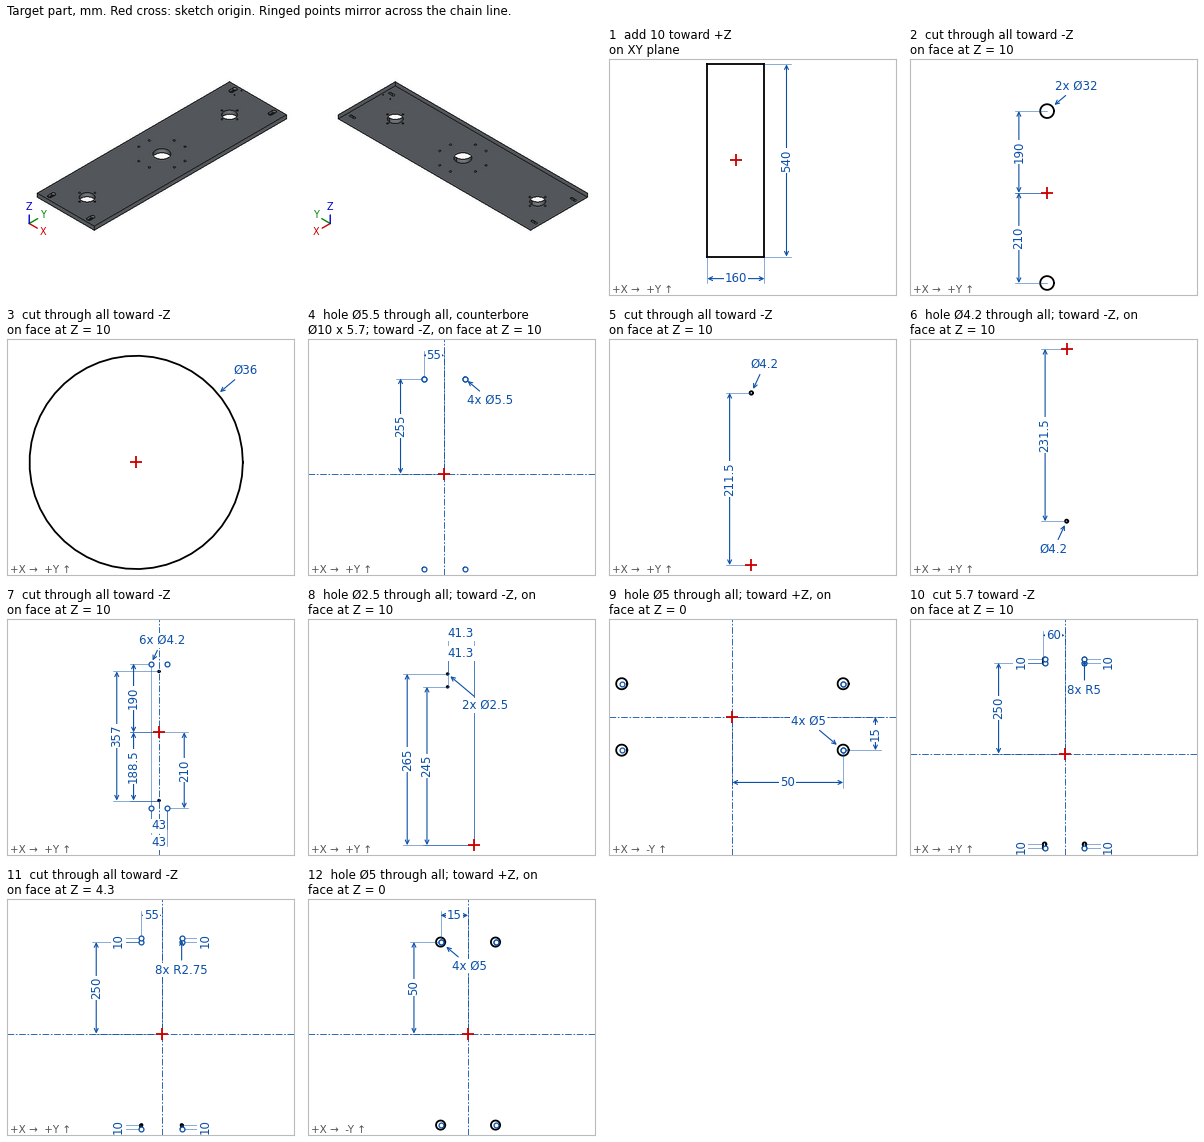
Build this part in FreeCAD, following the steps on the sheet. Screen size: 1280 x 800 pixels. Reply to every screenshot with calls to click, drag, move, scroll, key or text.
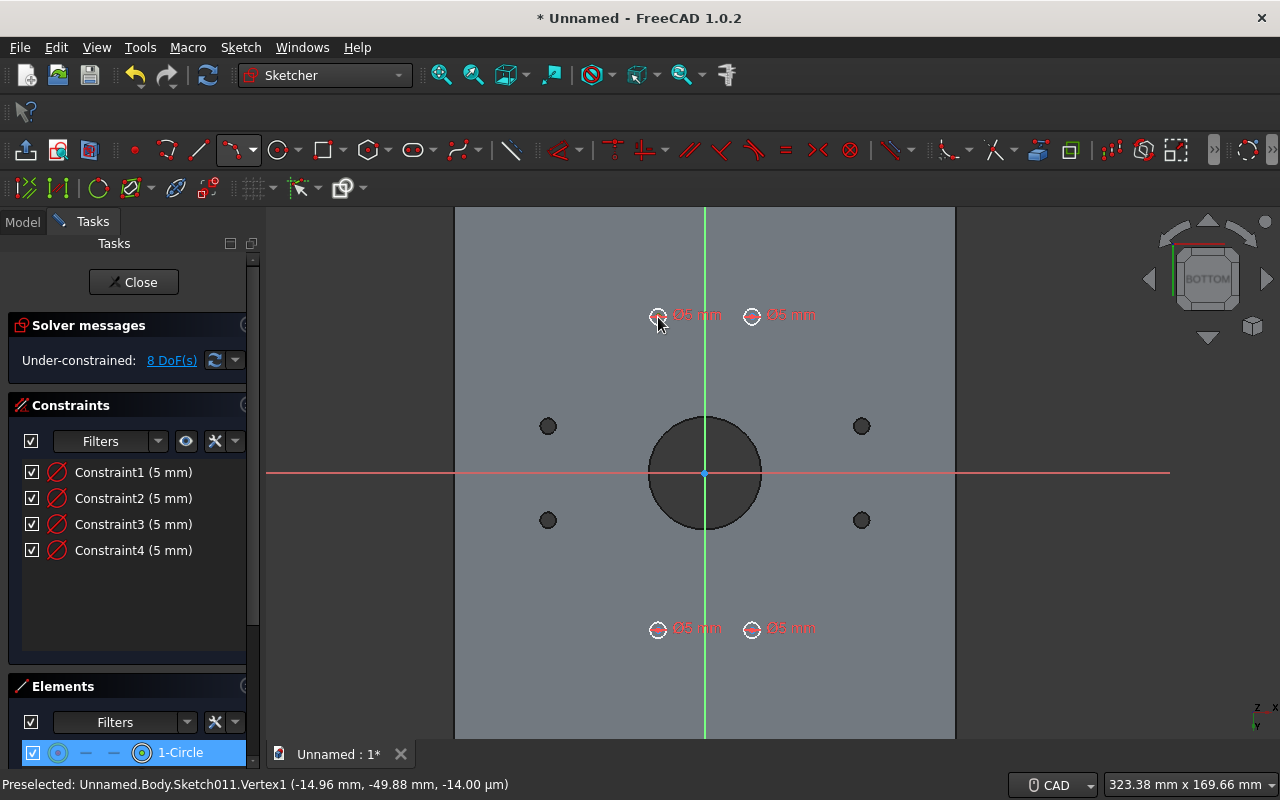
click(752, 317)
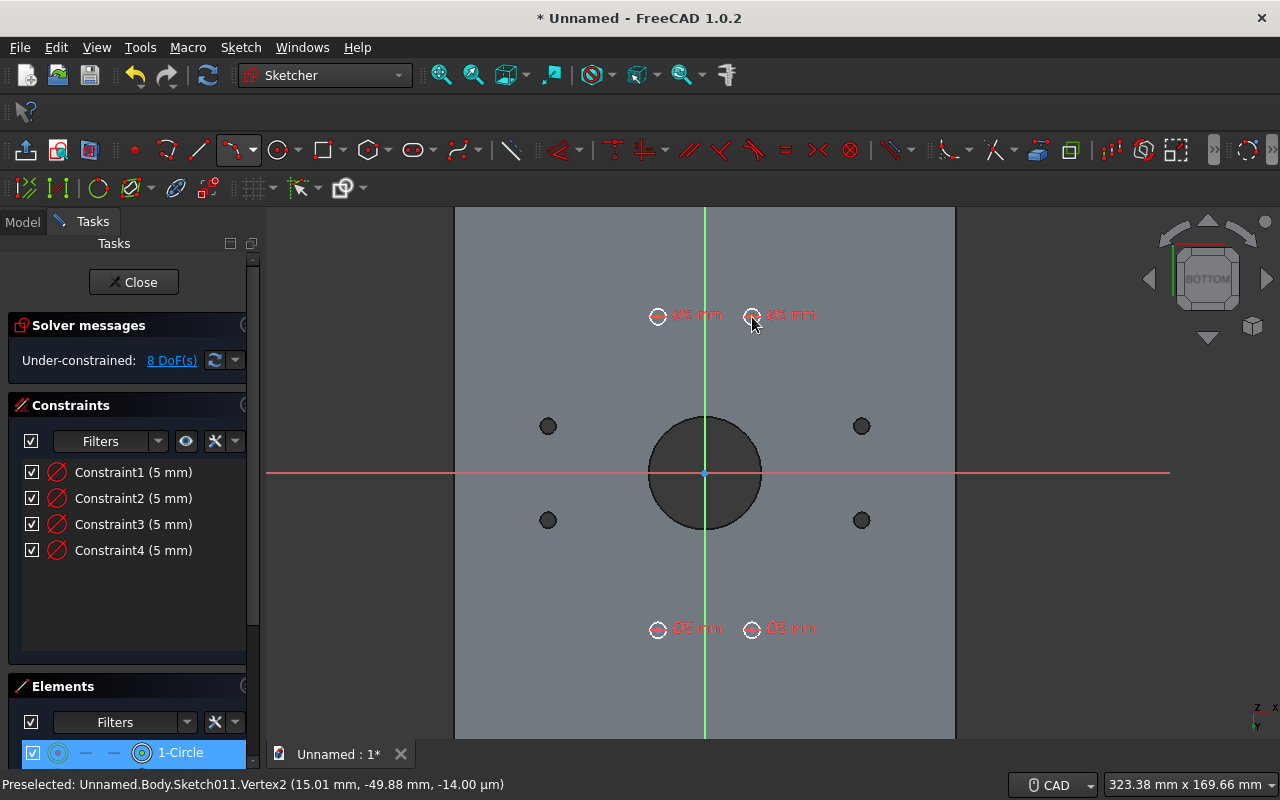
click(705, 677)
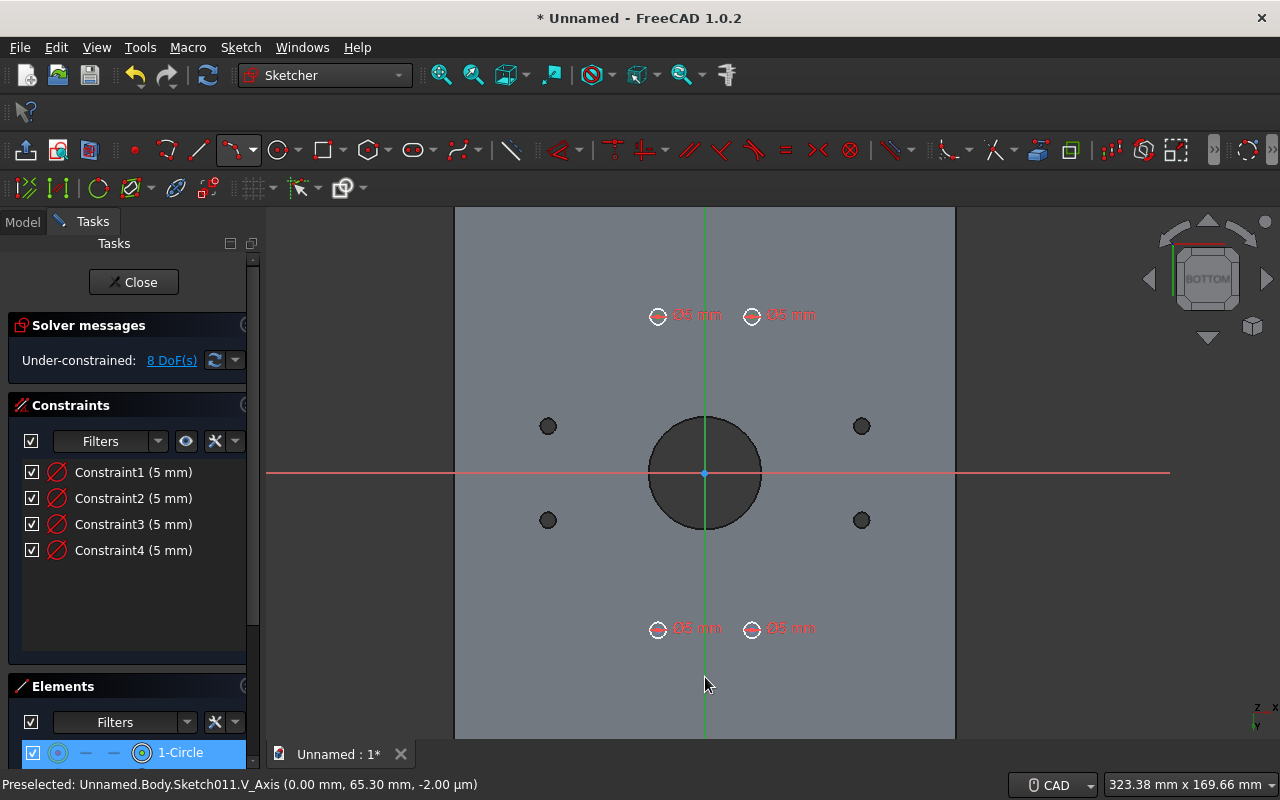
key(s)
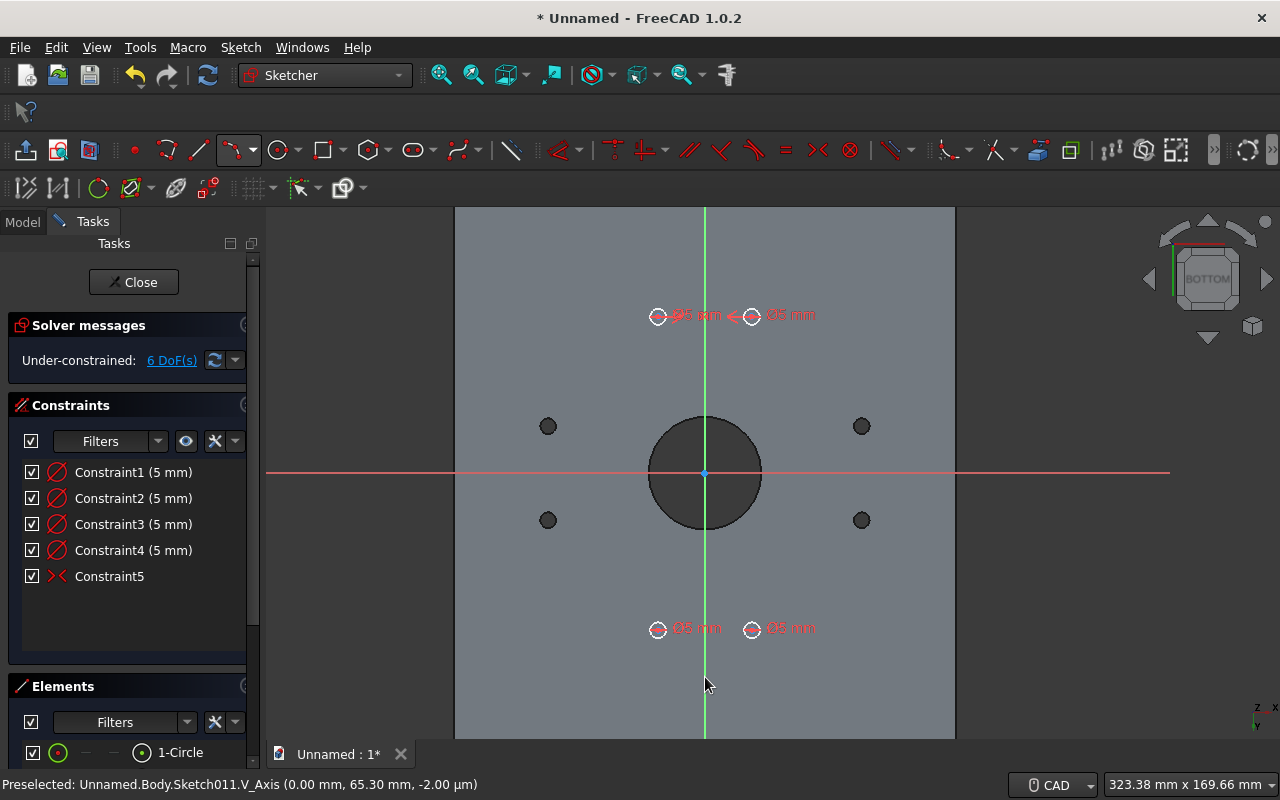
click(752, 317)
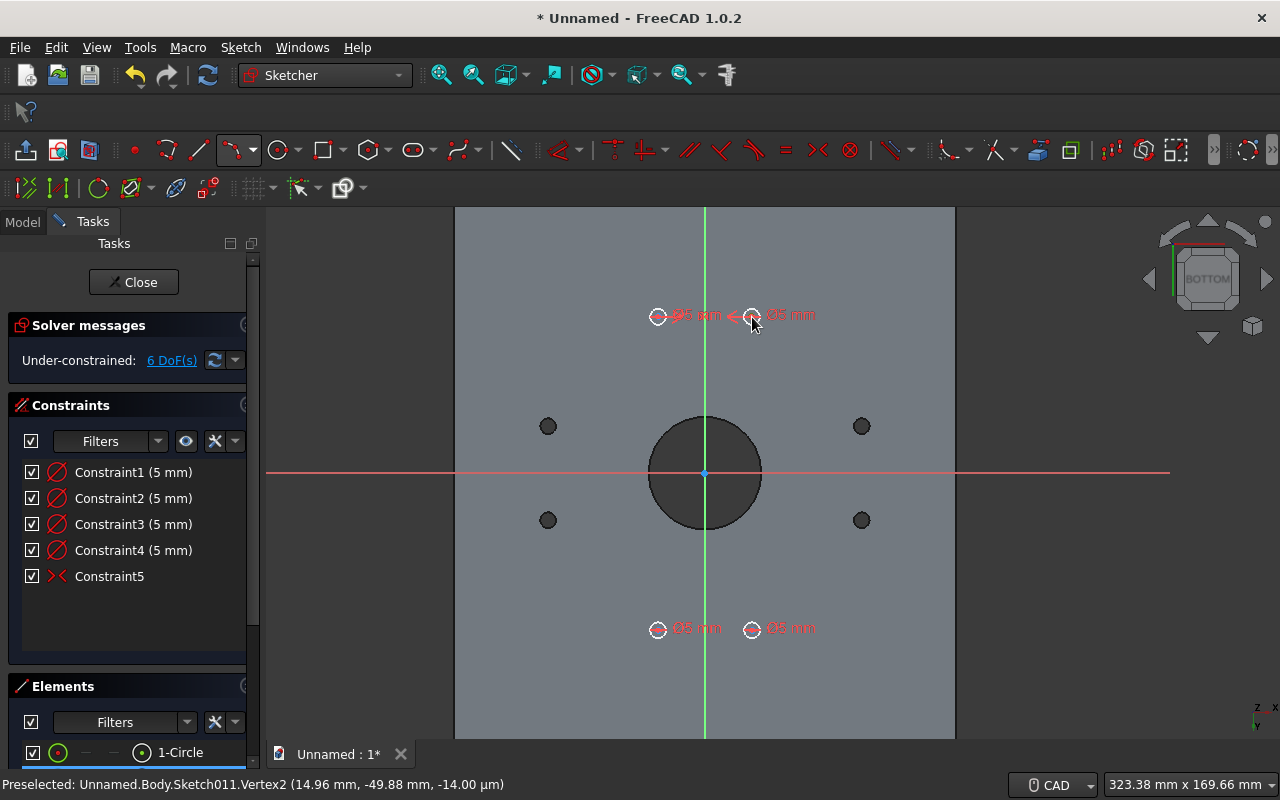
click(752, 630)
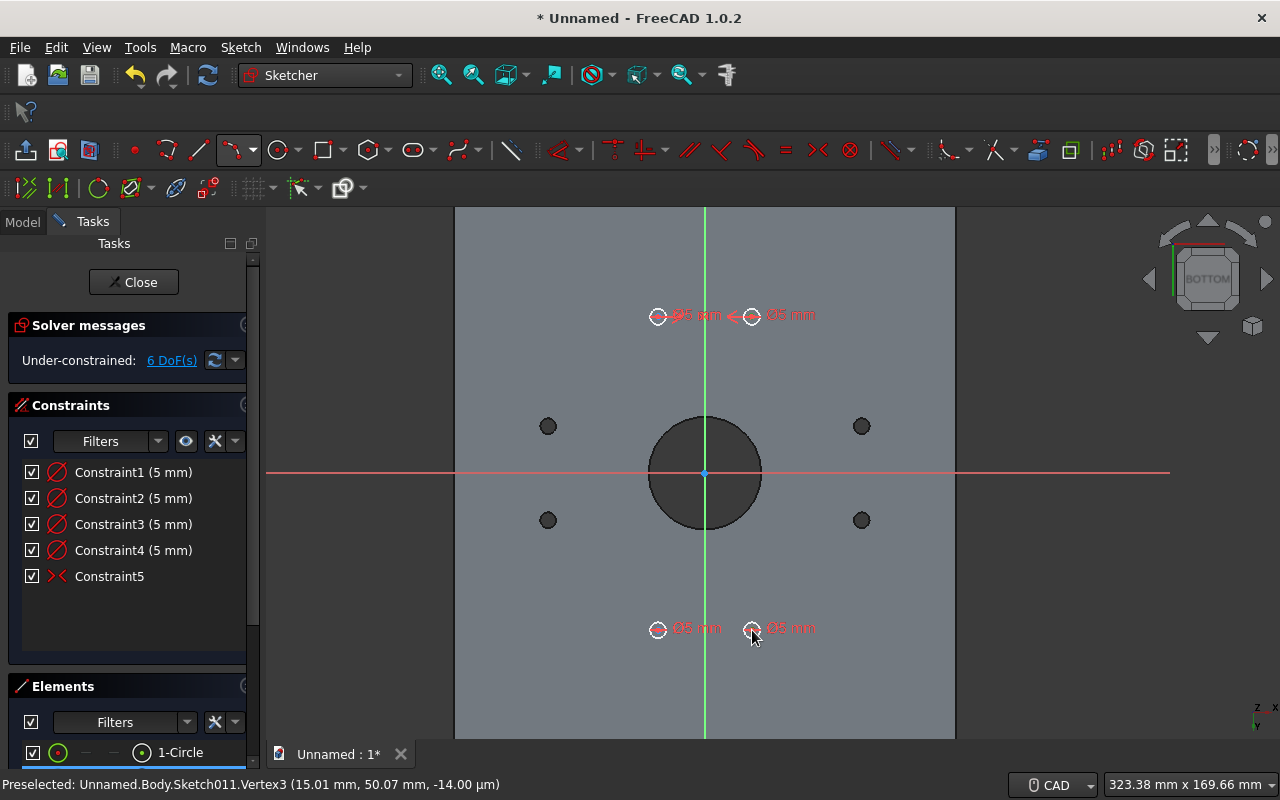
click(353, 473)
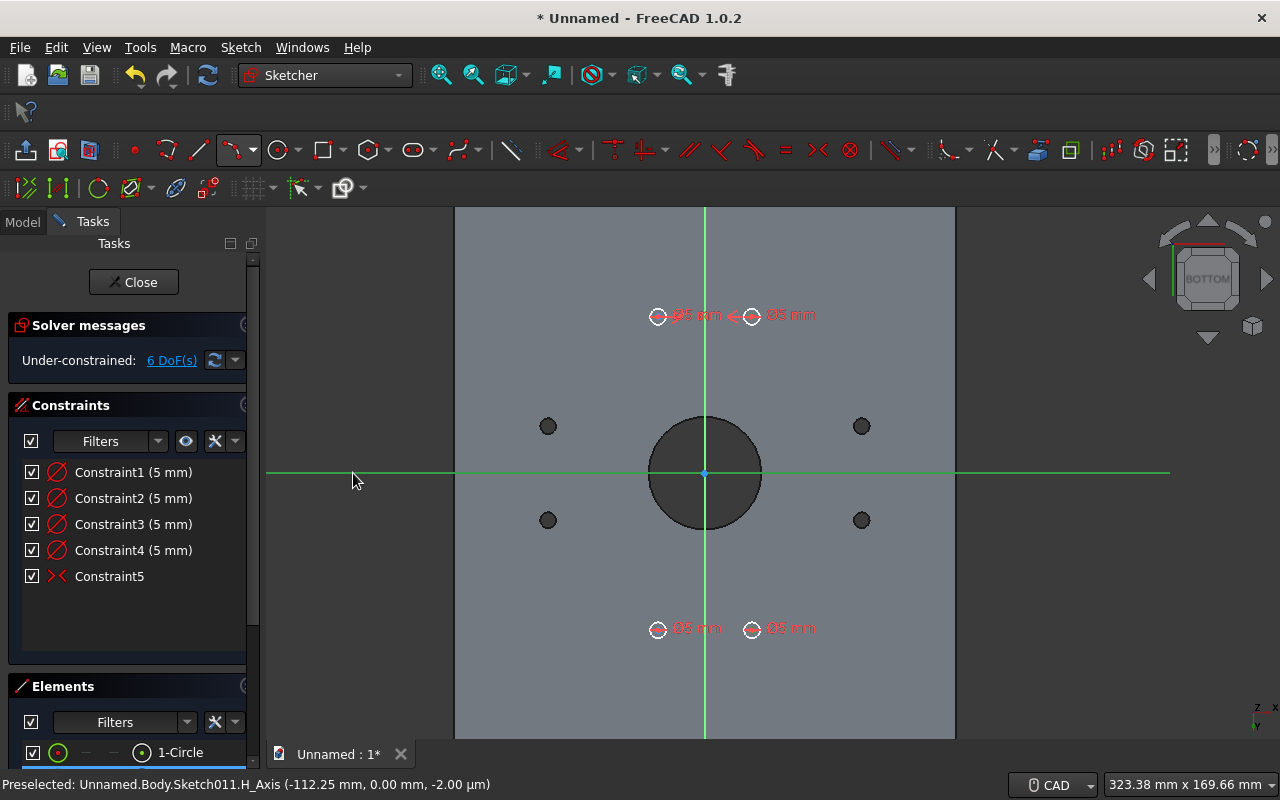
key(s)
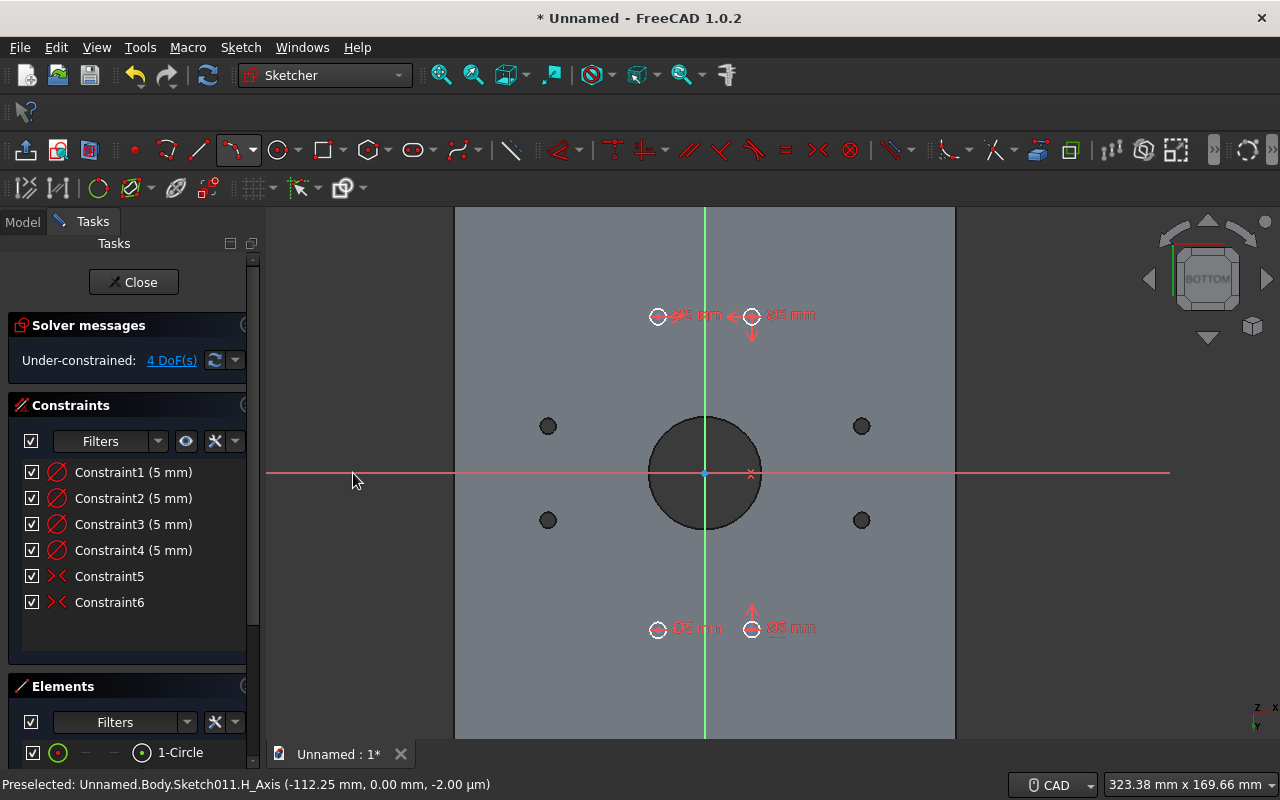
click(658, 317)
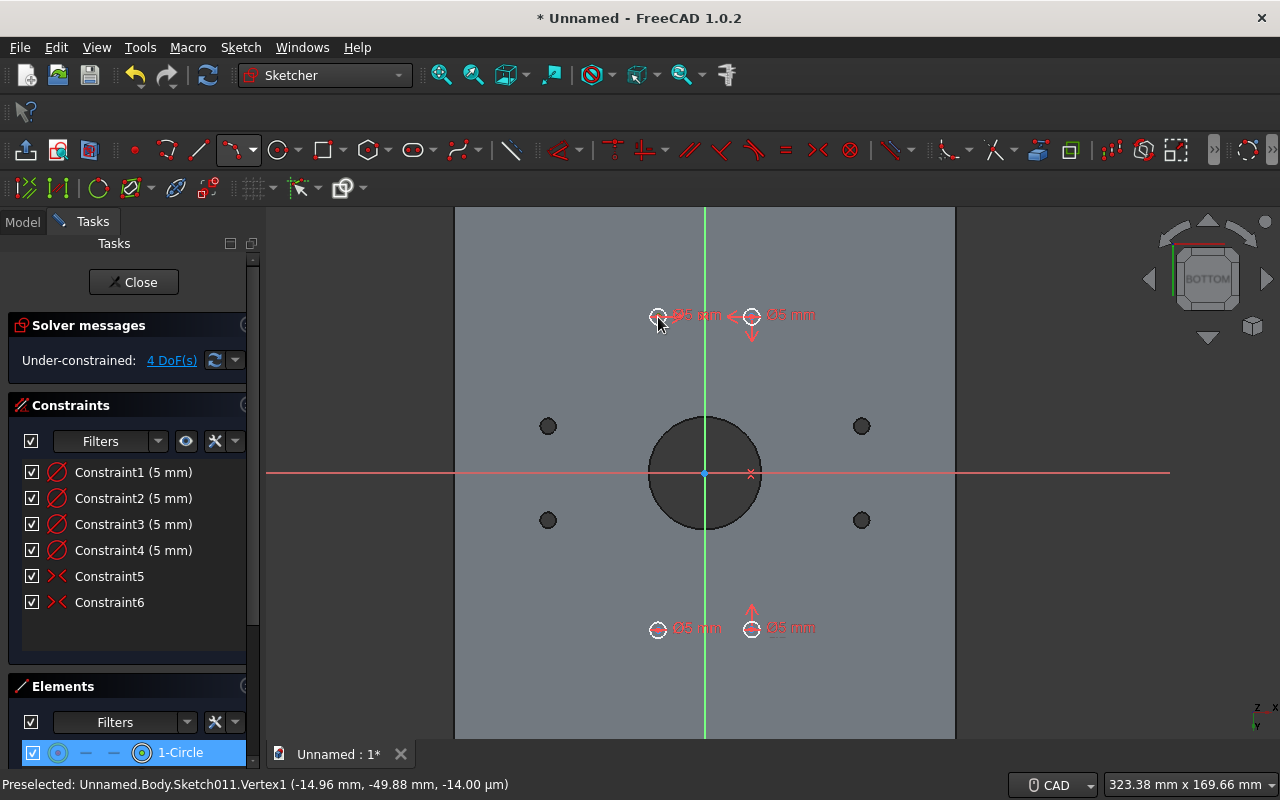
click(658, 630)